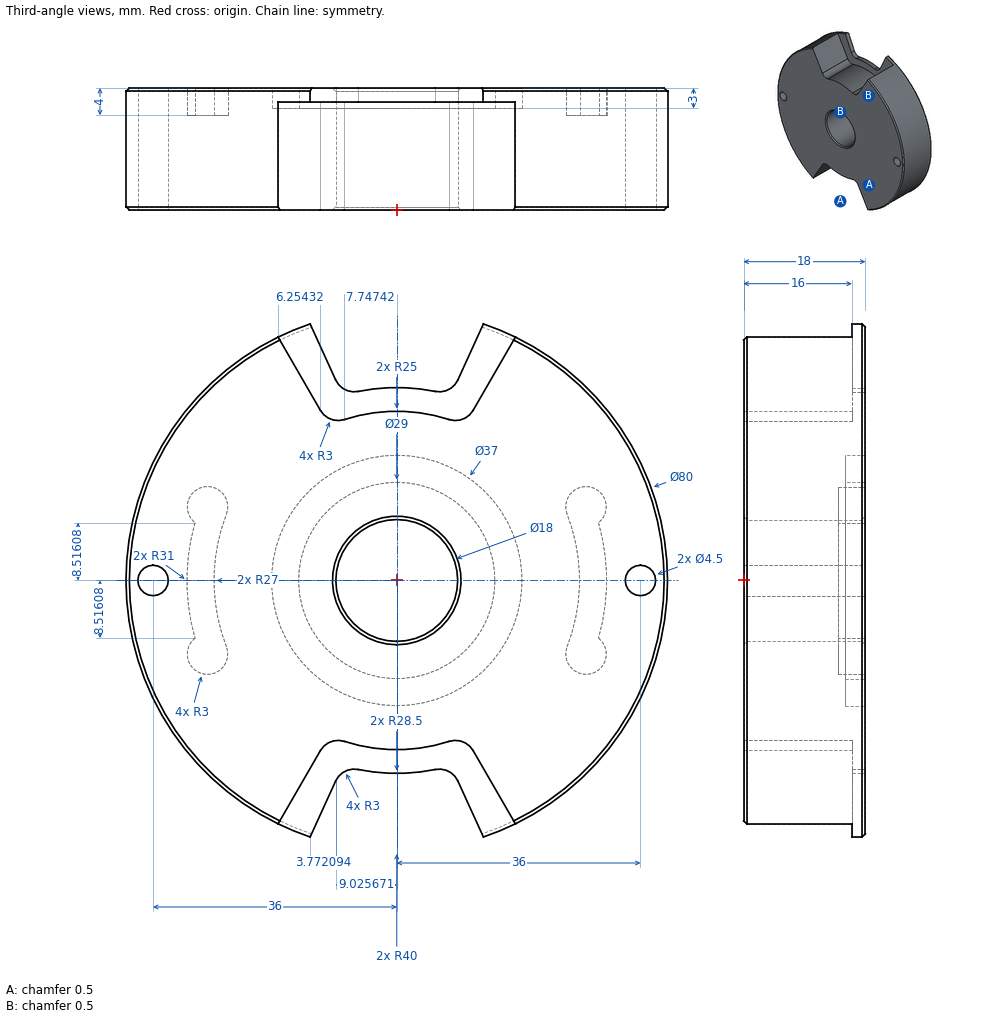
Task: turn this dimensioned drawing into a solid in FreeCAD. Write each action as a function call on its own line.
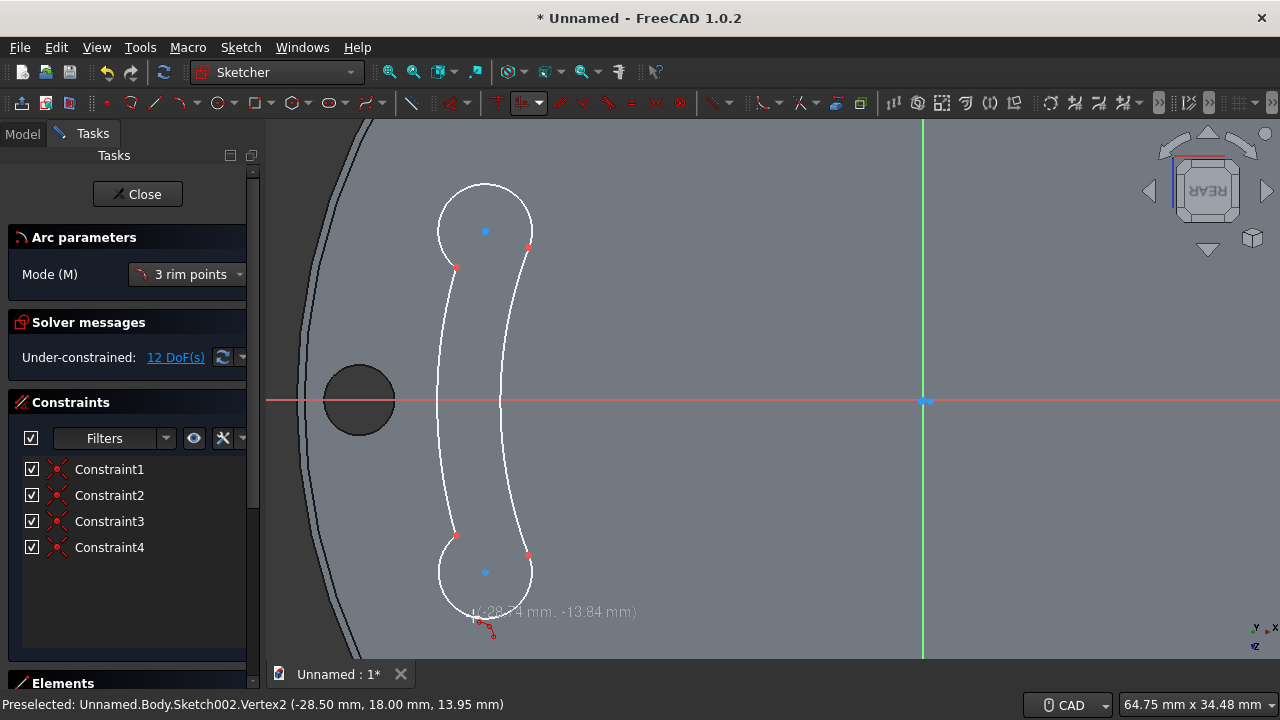
scroll(439, 375, down, 3)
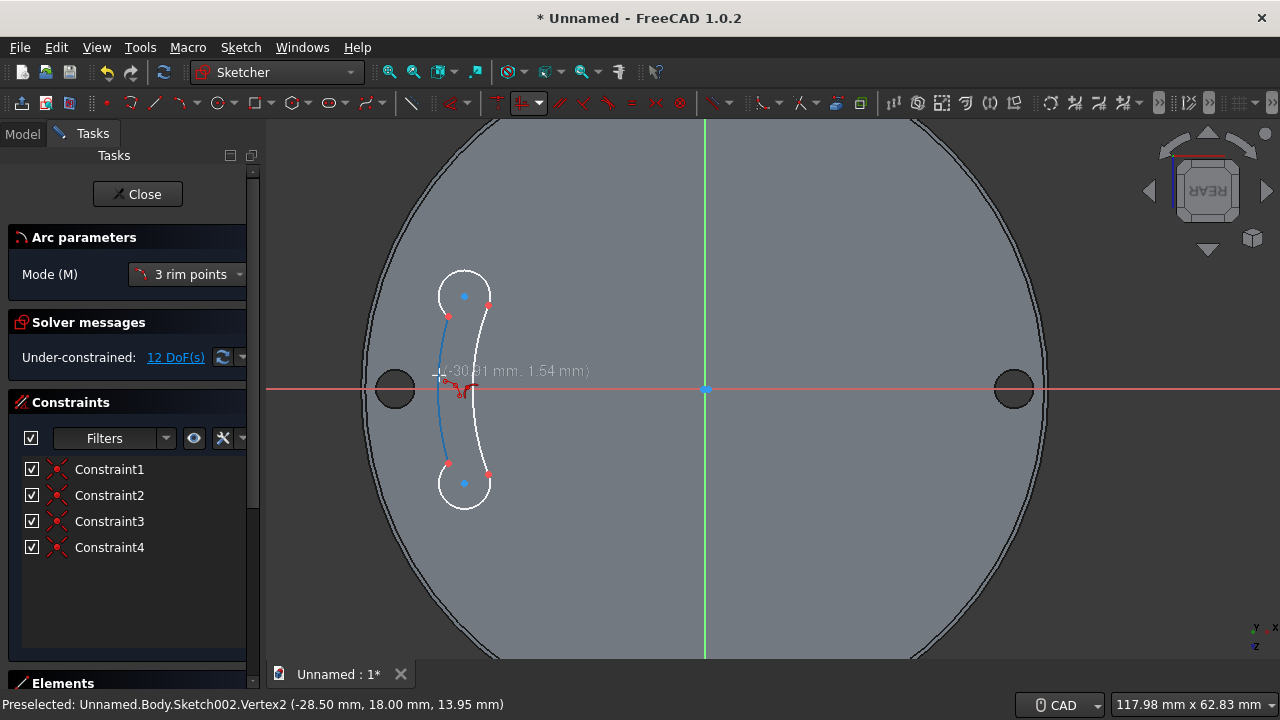
click(921, 473)
click(961, 462)
click(952, 507)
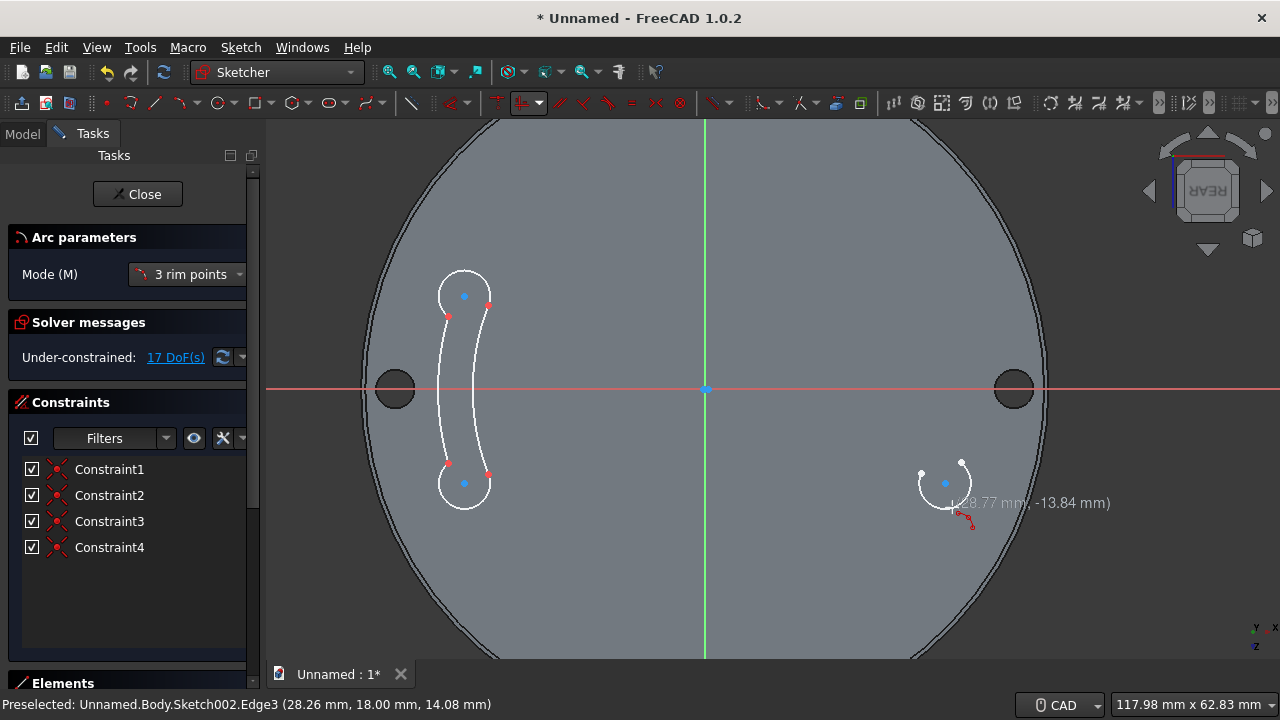
click(961, 463)
click(961, 316)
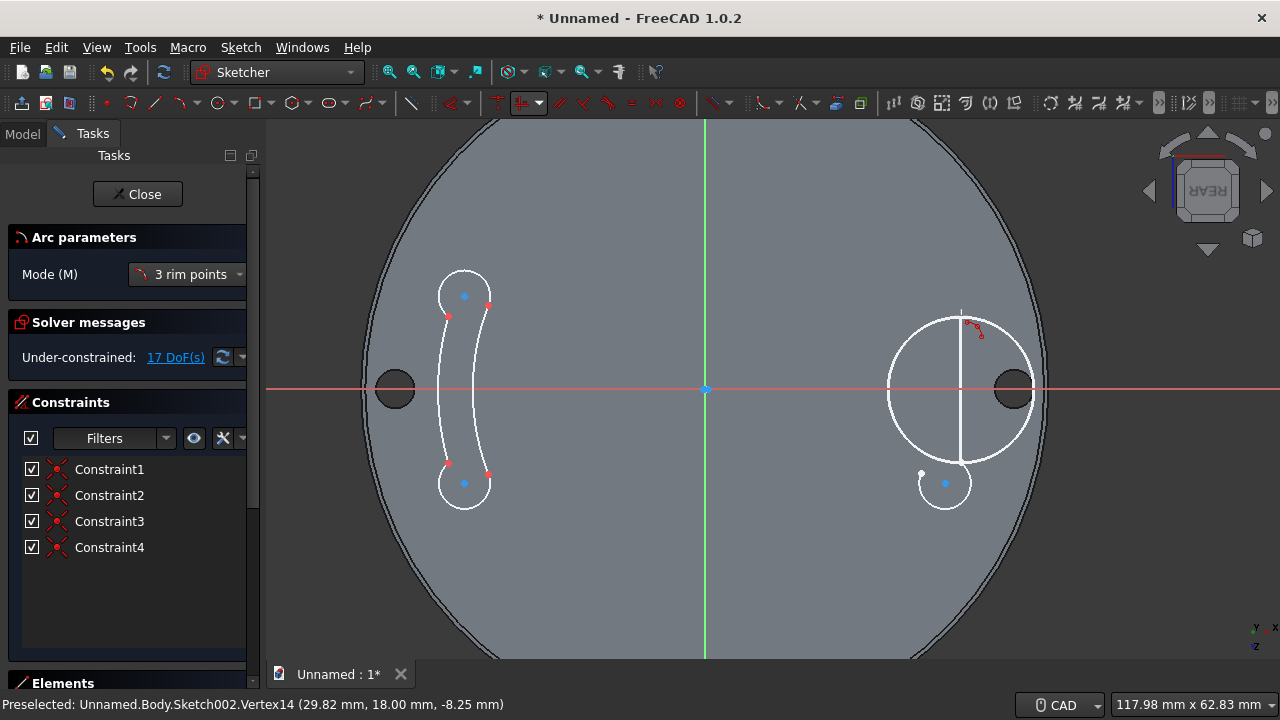
scroll(971, 404, up, 3)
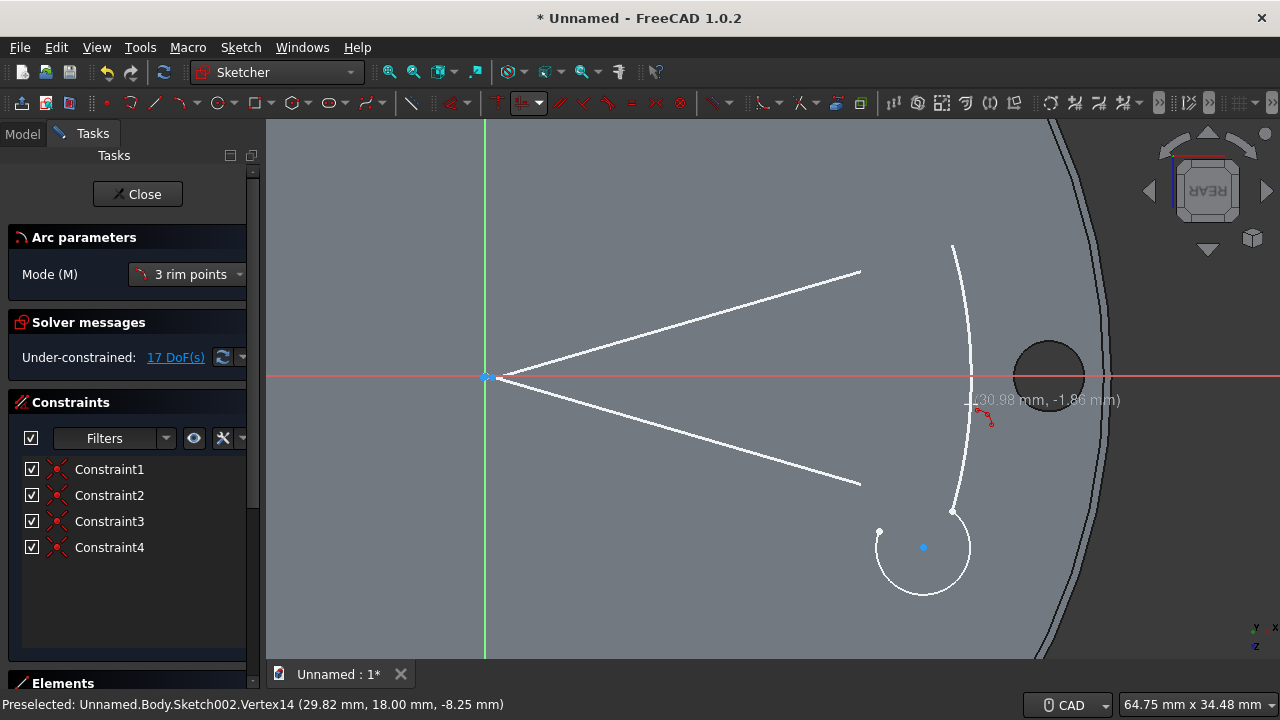
click(970, 403)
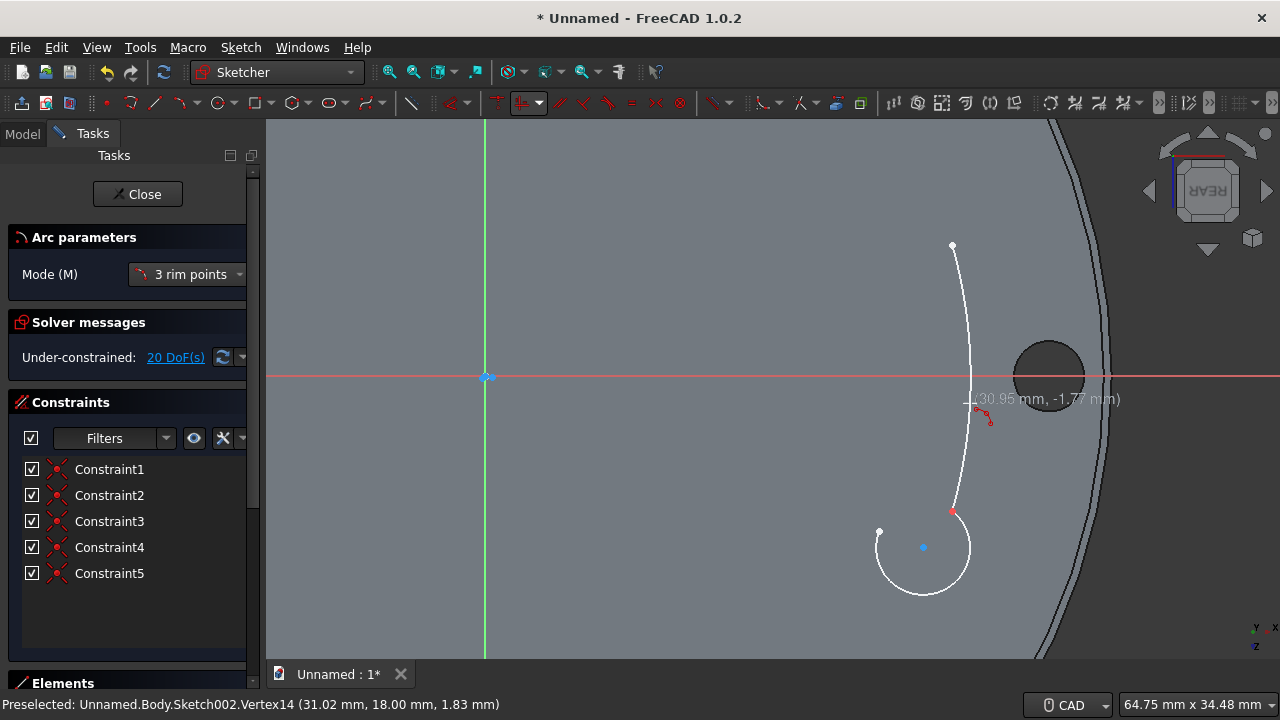
click(952, 245)
click(879, 223)
click(936, 161)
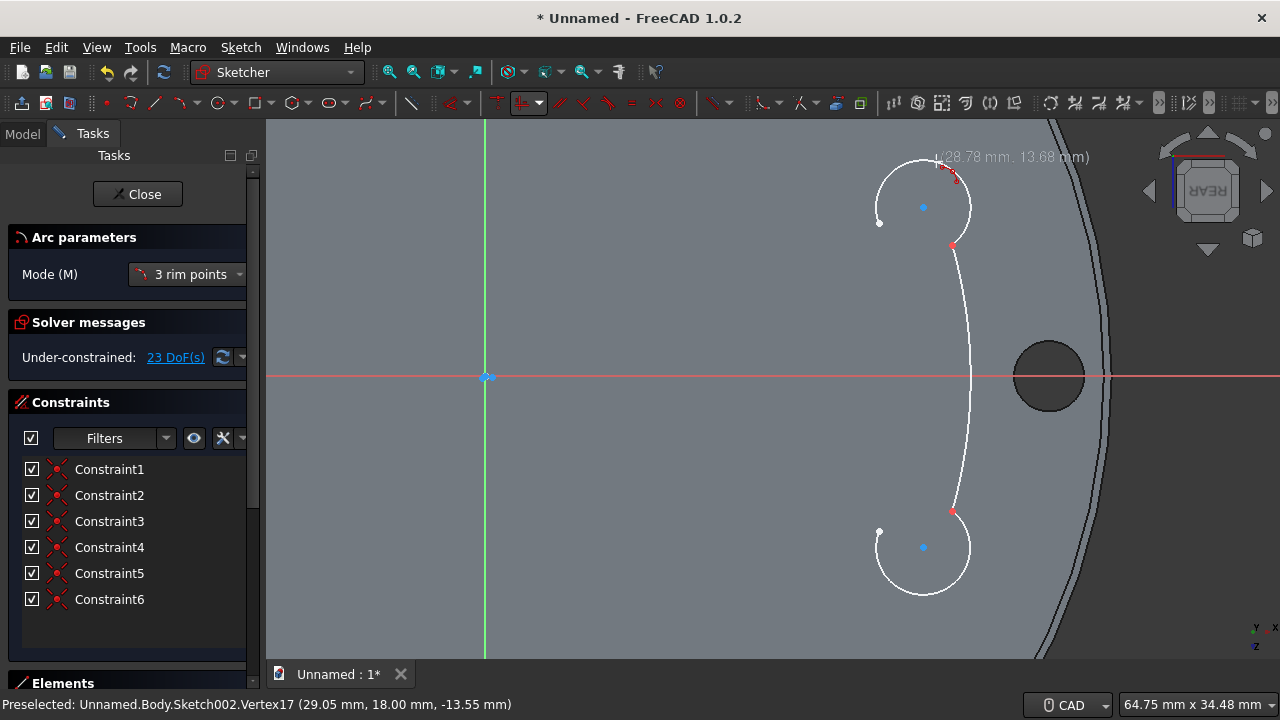
click(879, 224)
click(879, 531)
click(907, 408)
key(Escape)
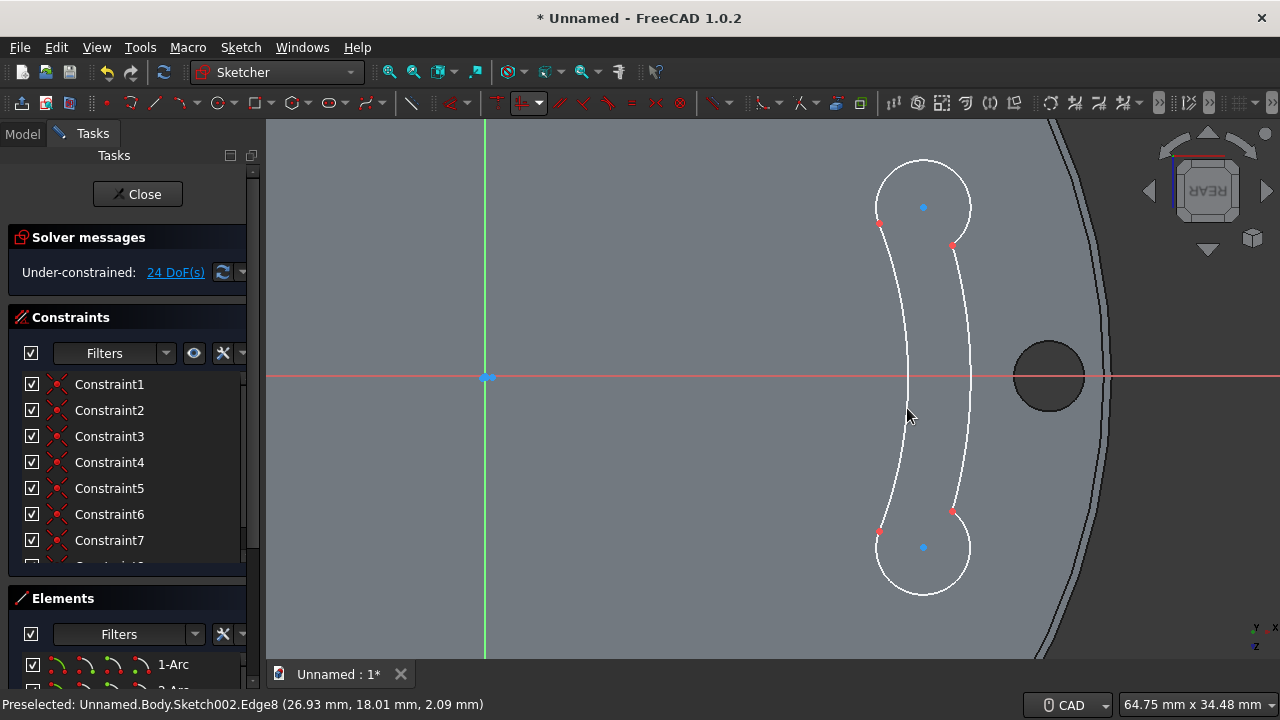
scroll(971, 404, down, 3)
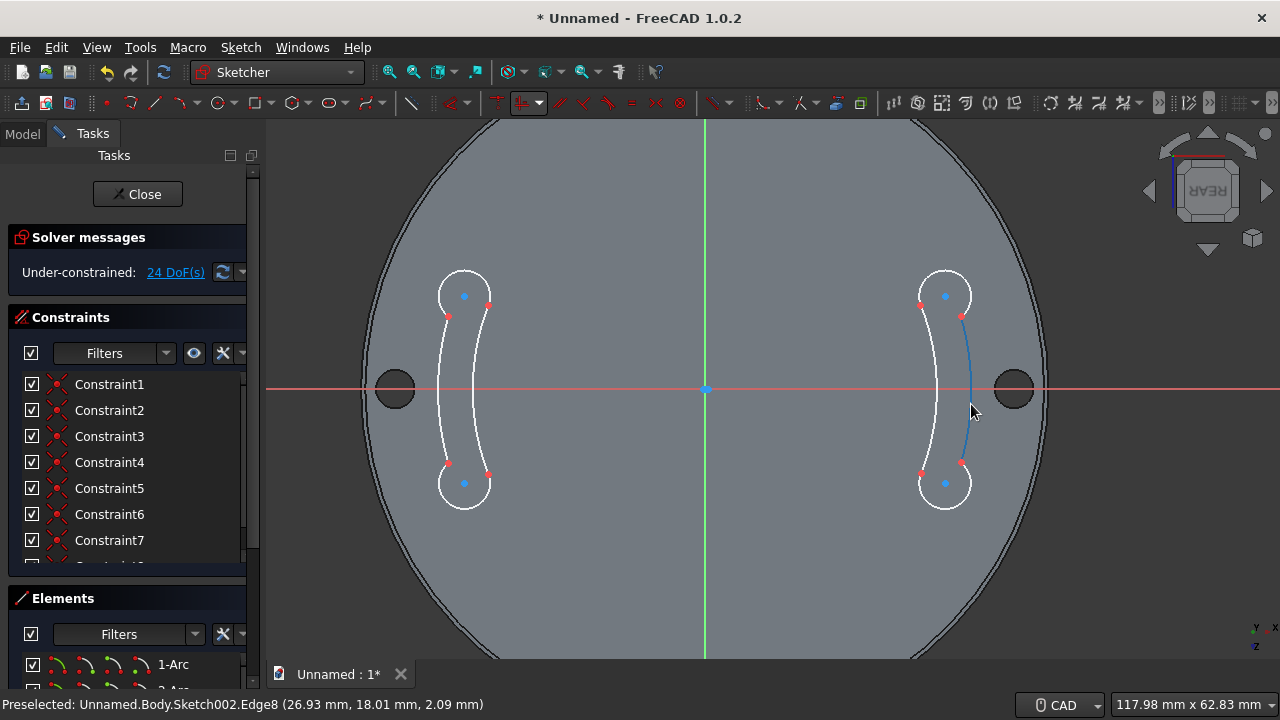
click(475, 356)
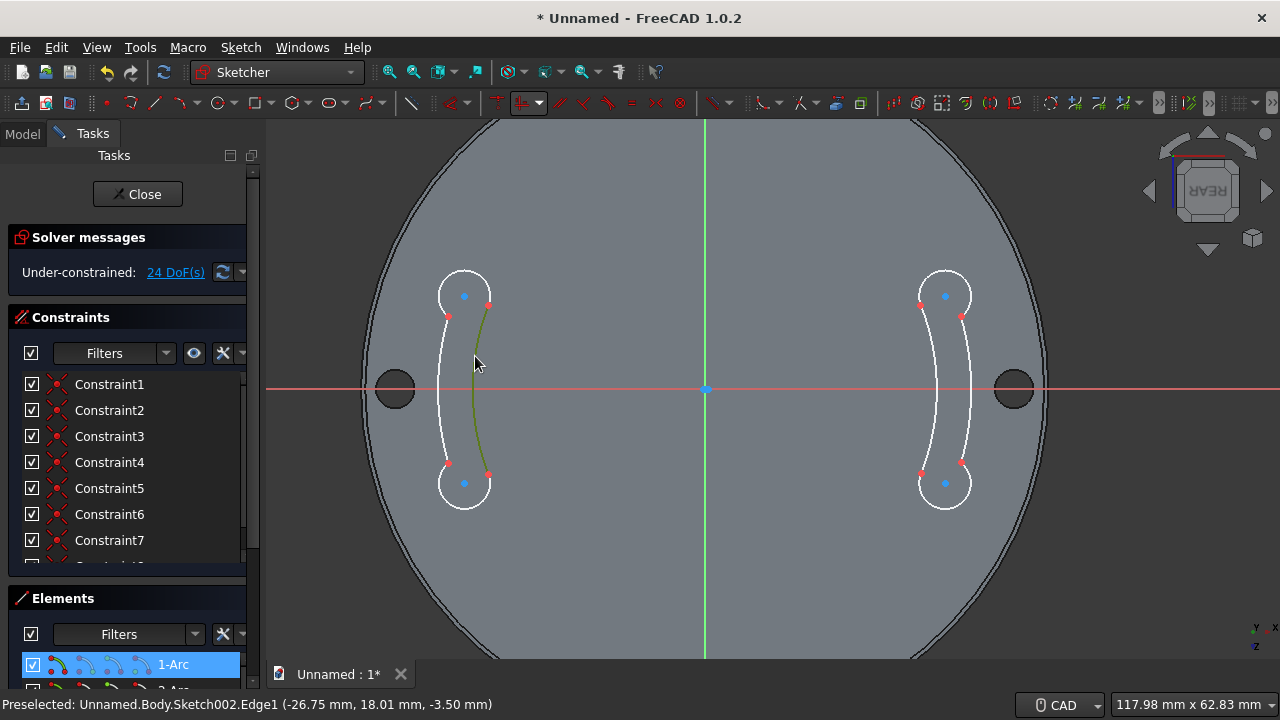
click(479, 275)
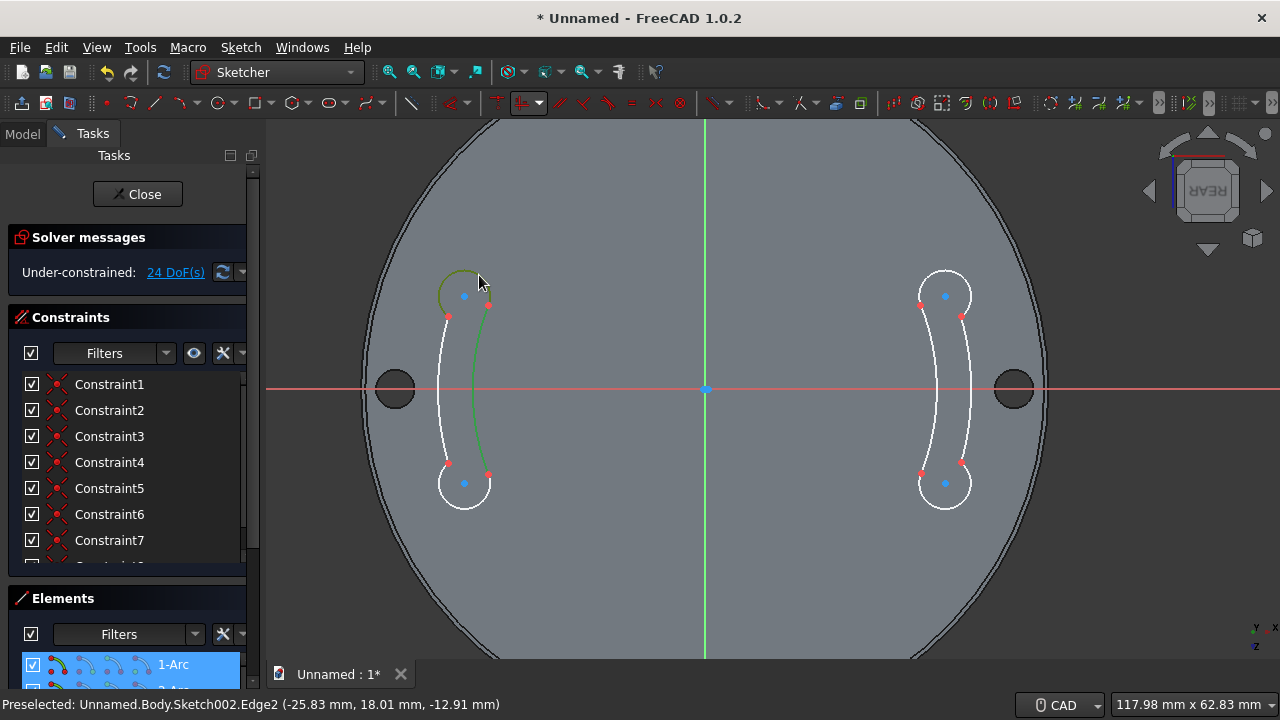
click(608, 104)